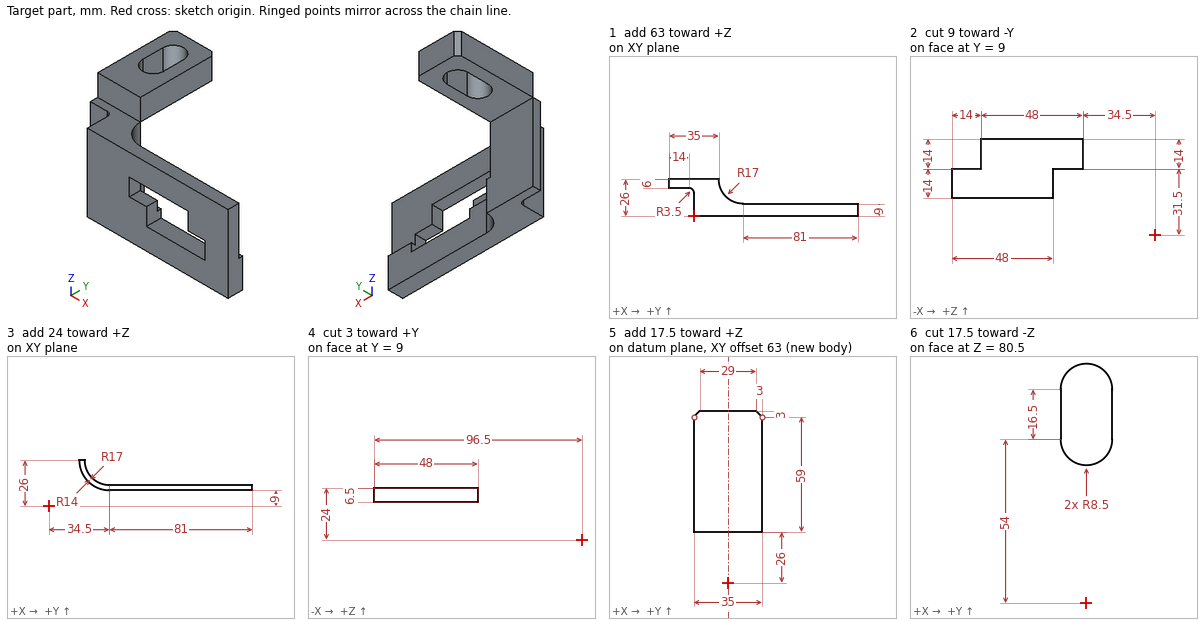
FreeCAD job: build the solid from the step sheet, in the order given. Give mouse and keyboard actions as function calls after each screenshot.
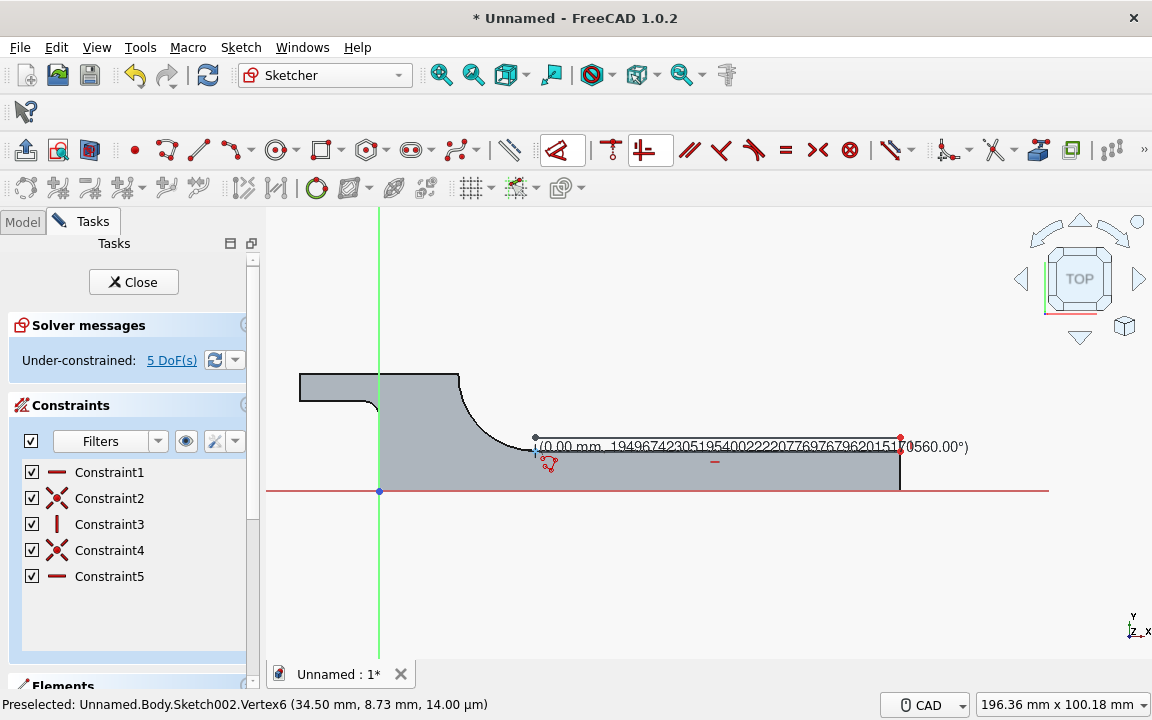
key(g)
key(l)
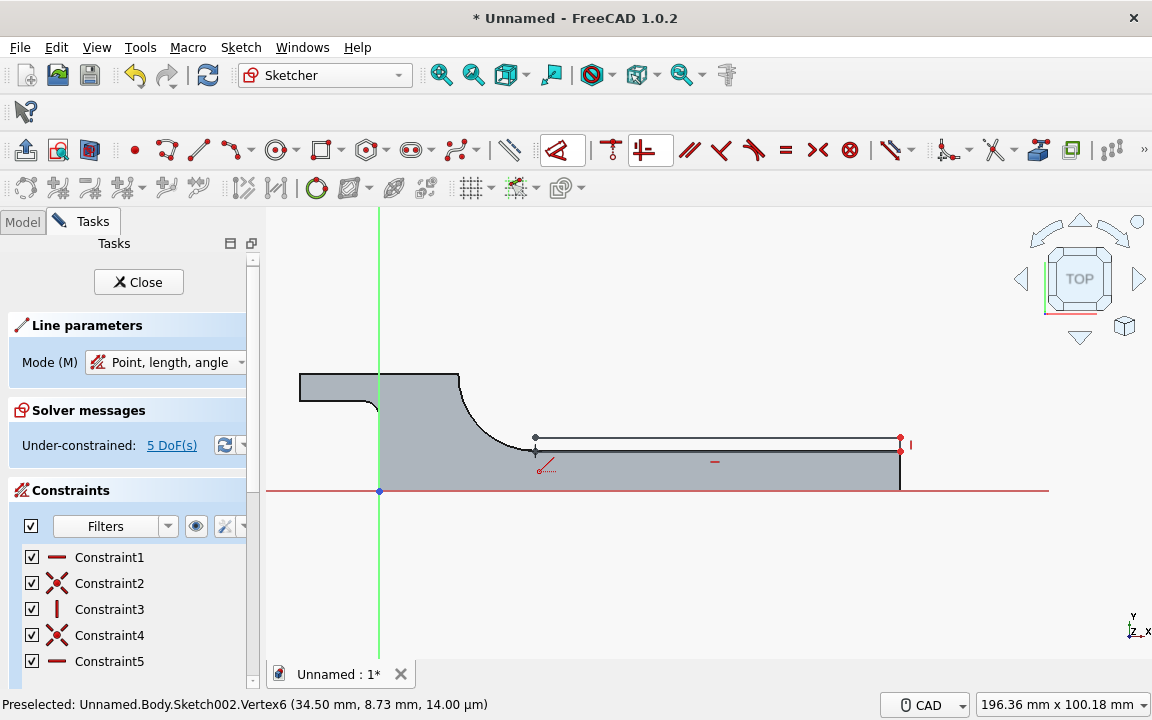
click(458, 374)
click(472, 374)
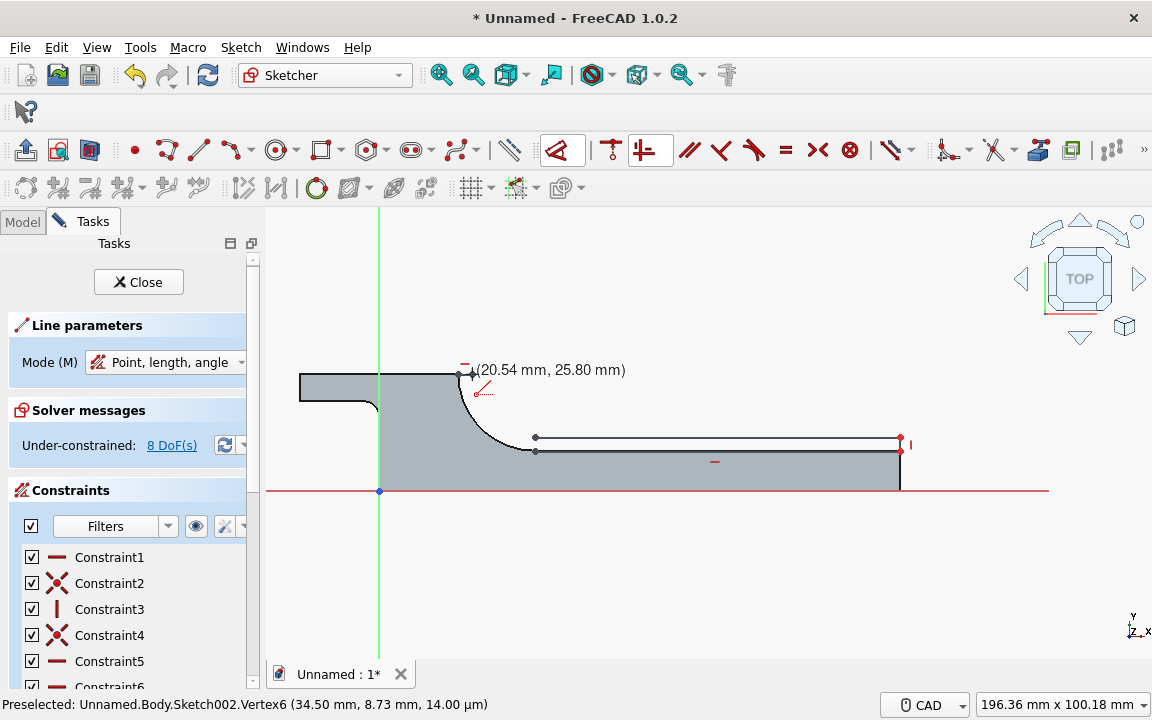
click(232, 150)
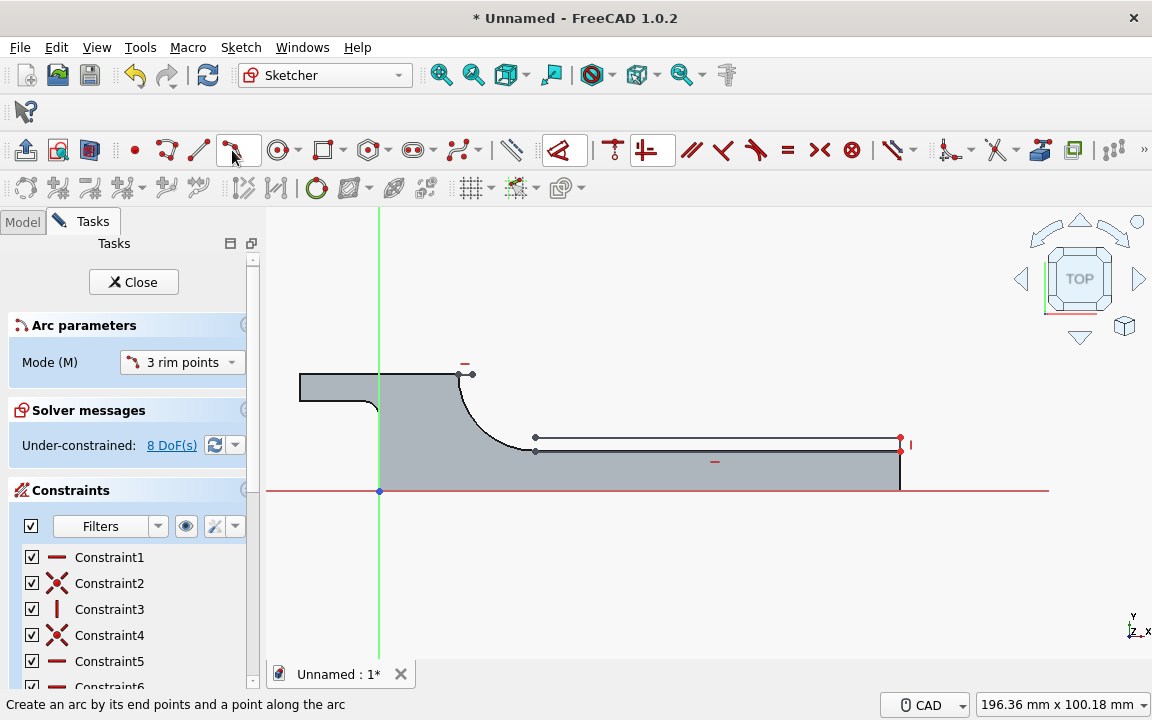
click(535, 452)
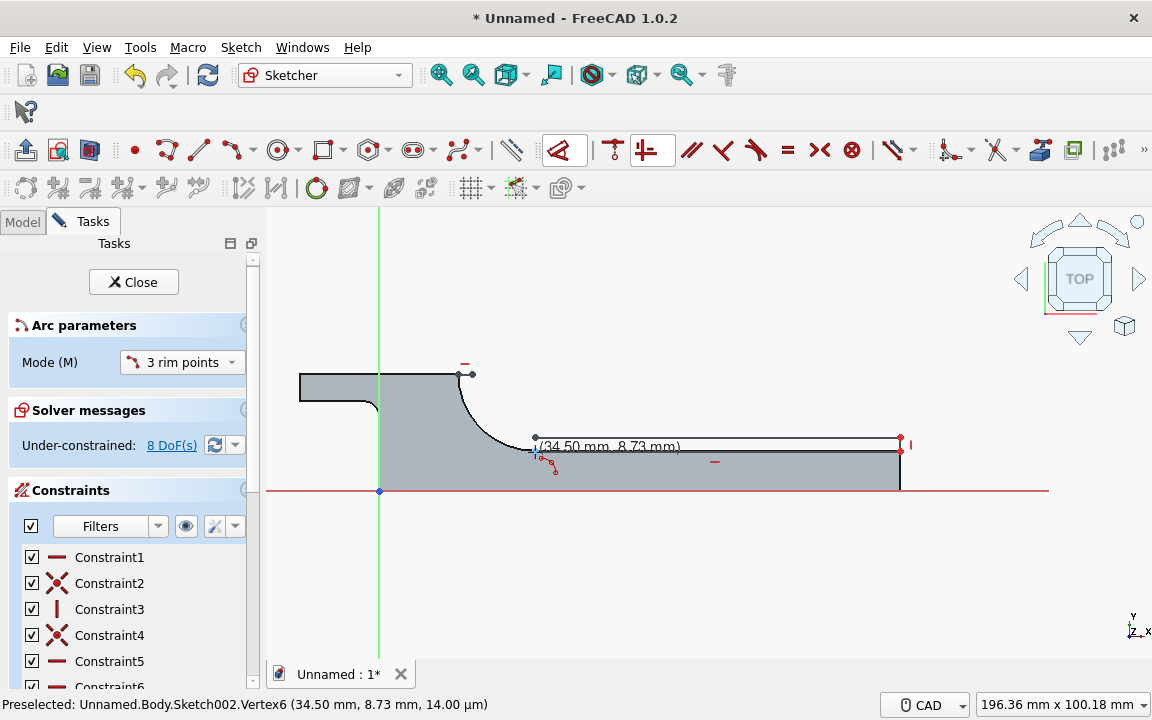
scroll(458, 374, up, 5)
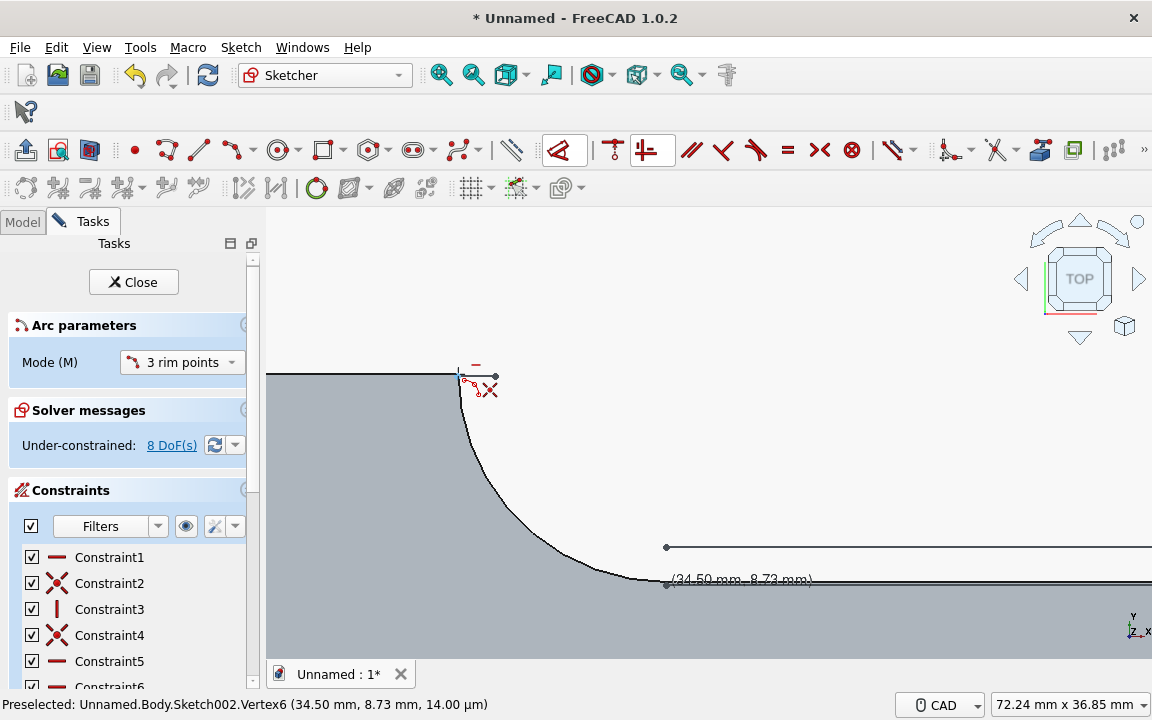
click(458, 376)
click(520, 521)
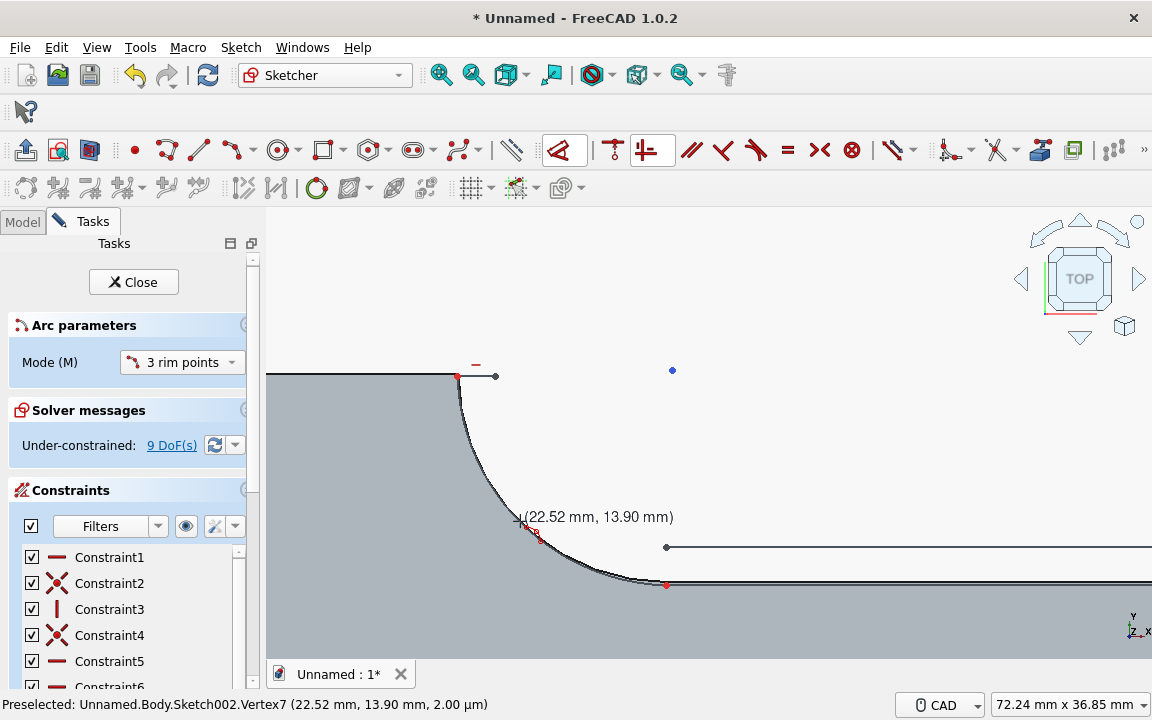
click(496, 376)
click(667, 547)
click(546, 495)
key(Escape)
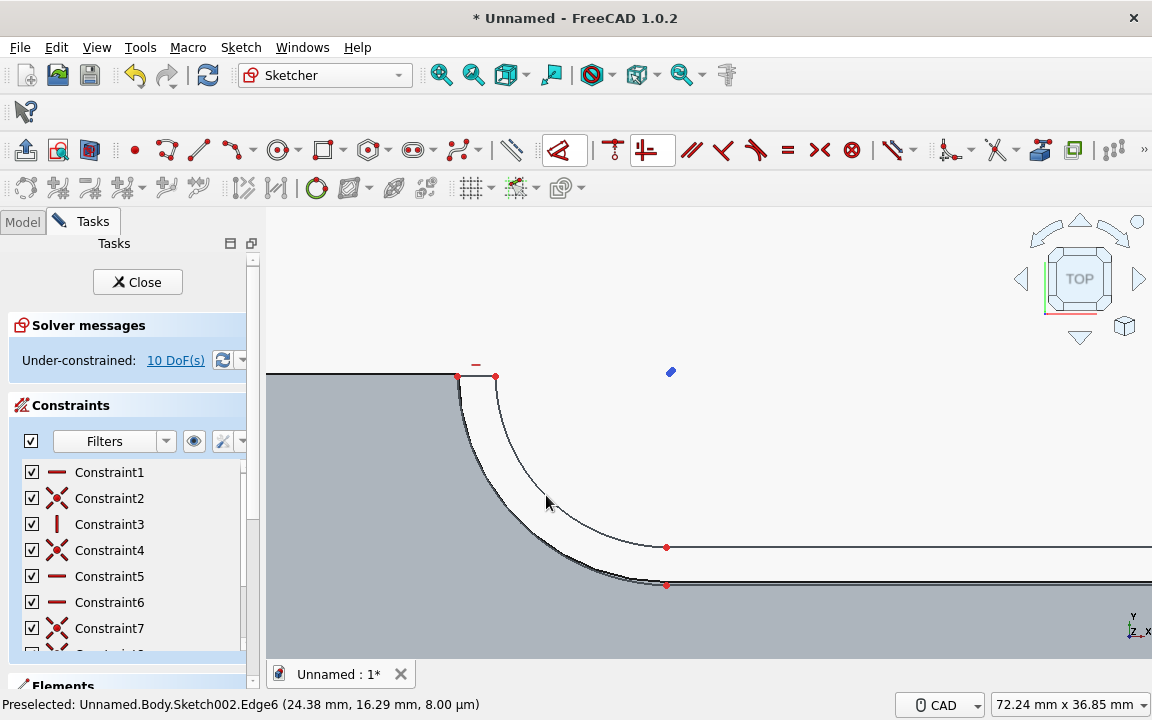
click(965, 547)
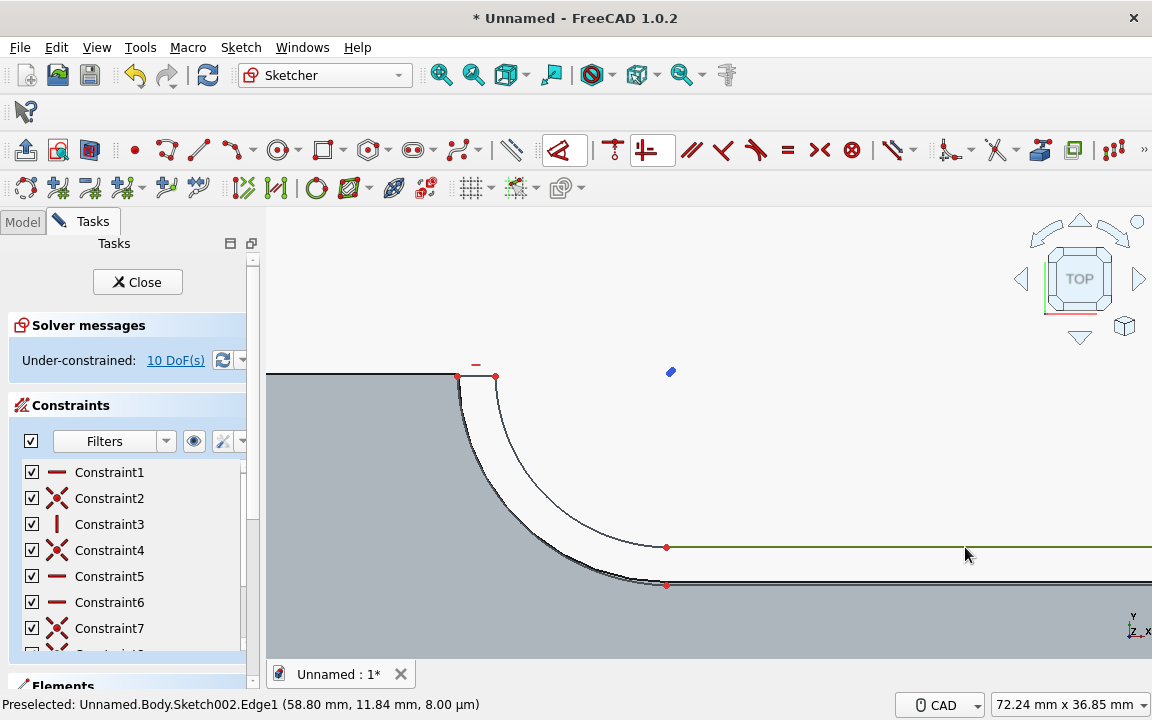
click(515, 453)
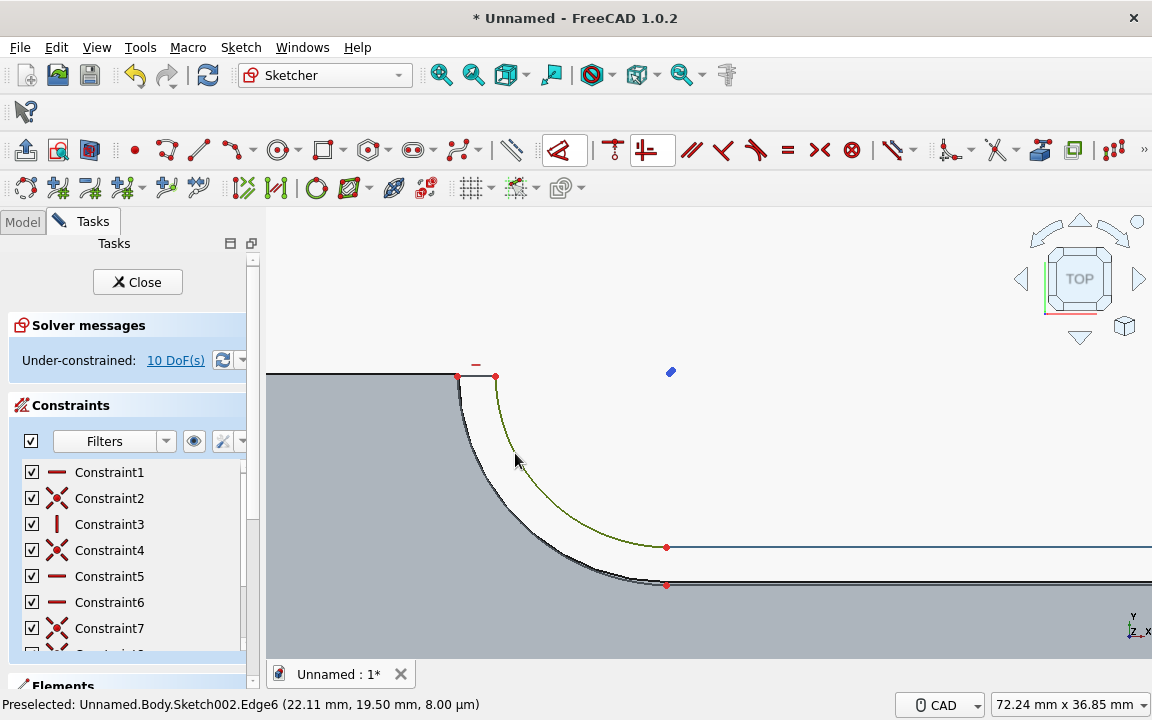
click(756, 150)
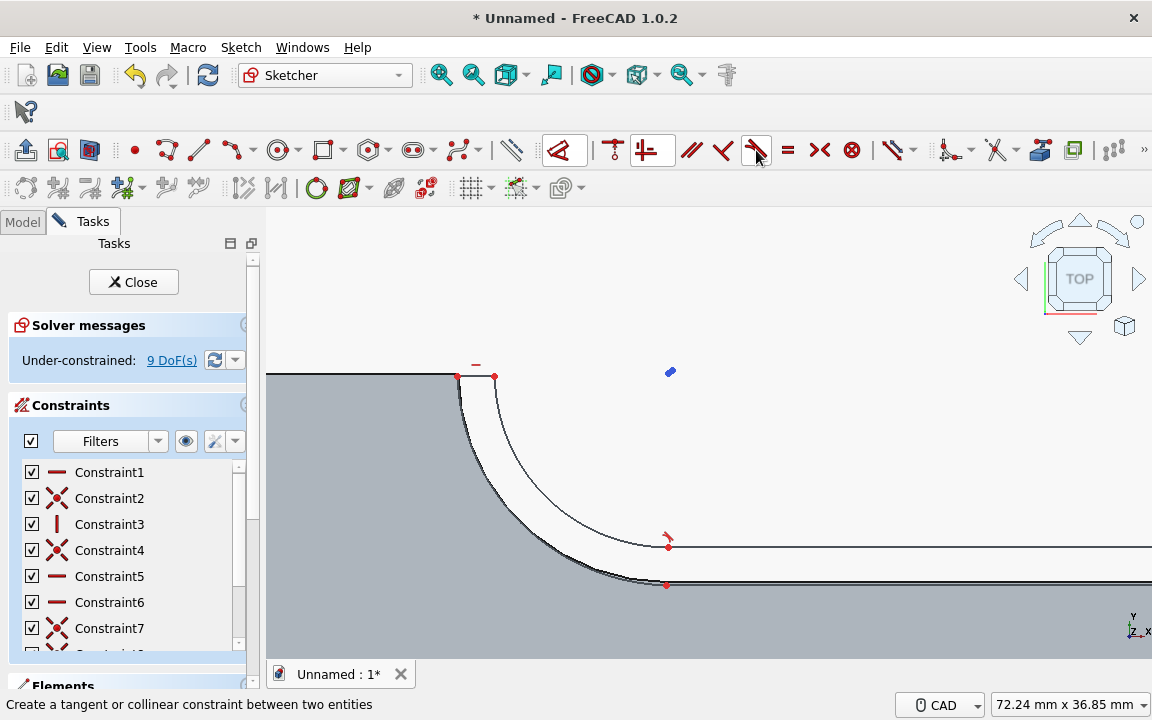
click(965, 585)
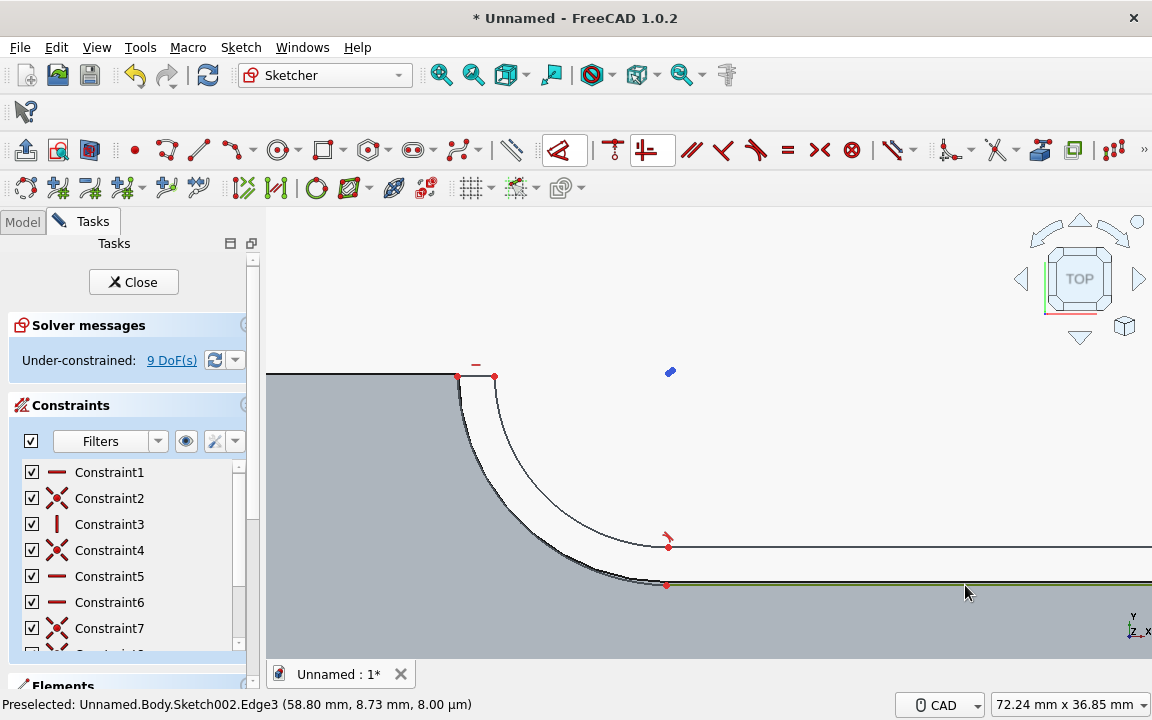
click(482, 470)